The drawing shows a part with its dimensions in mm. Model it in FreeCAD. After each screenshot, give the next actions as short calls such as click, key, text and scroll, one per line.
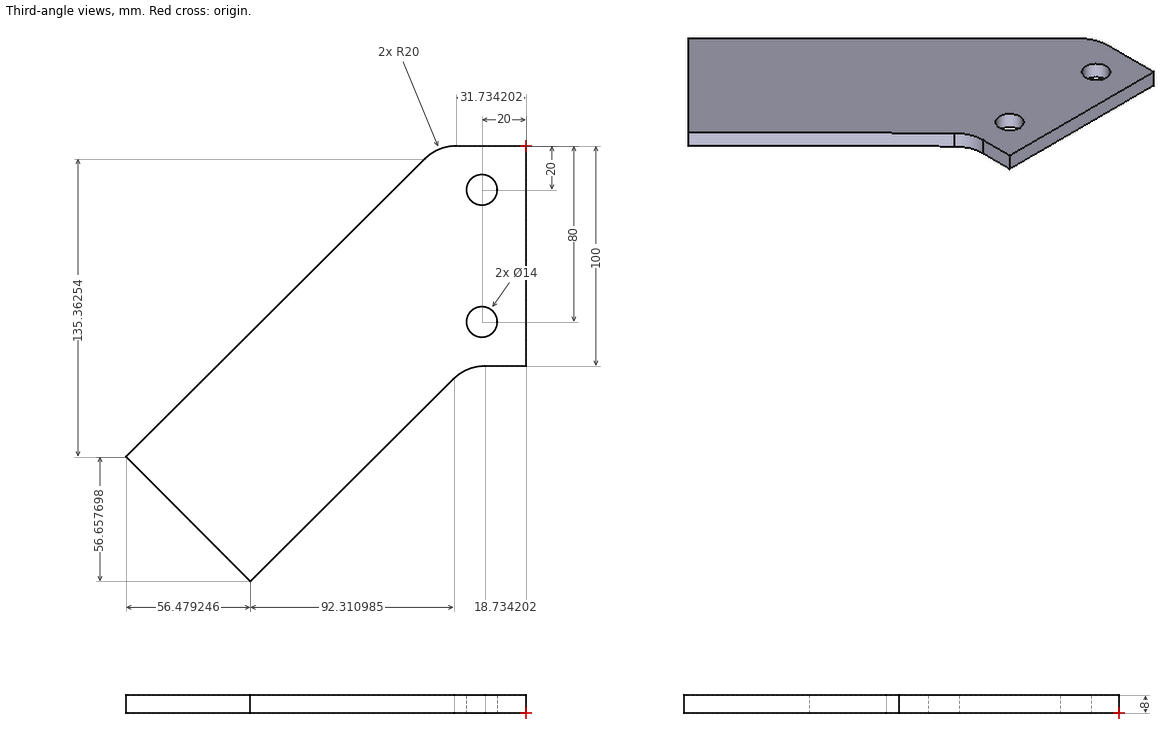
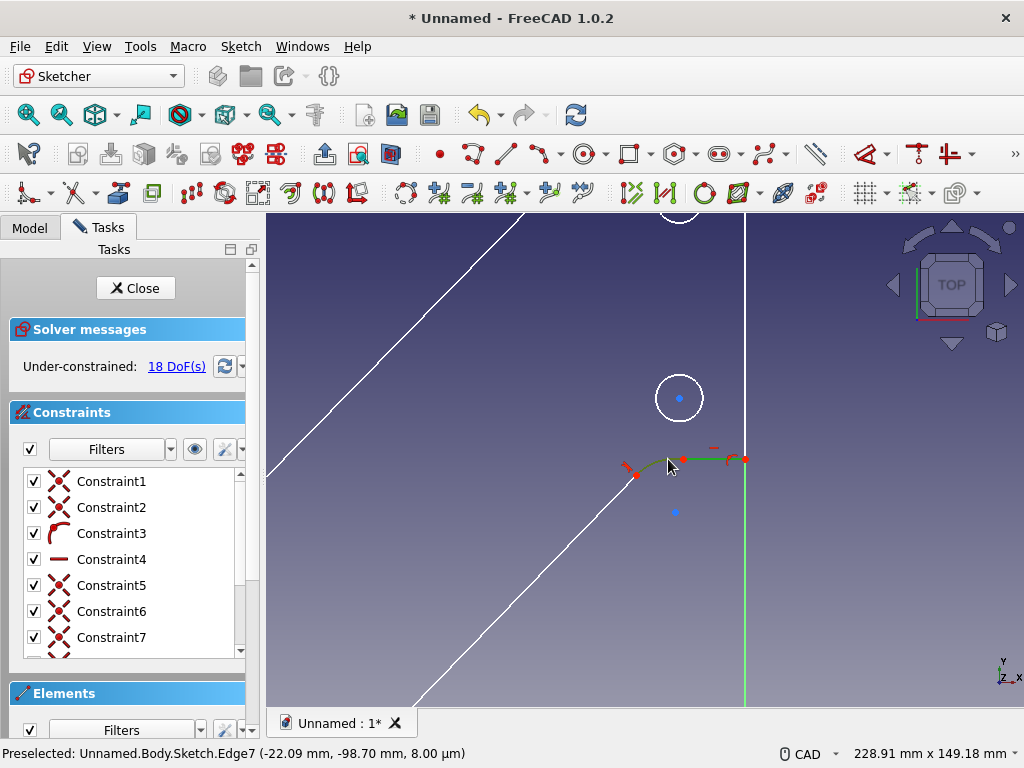
key(t)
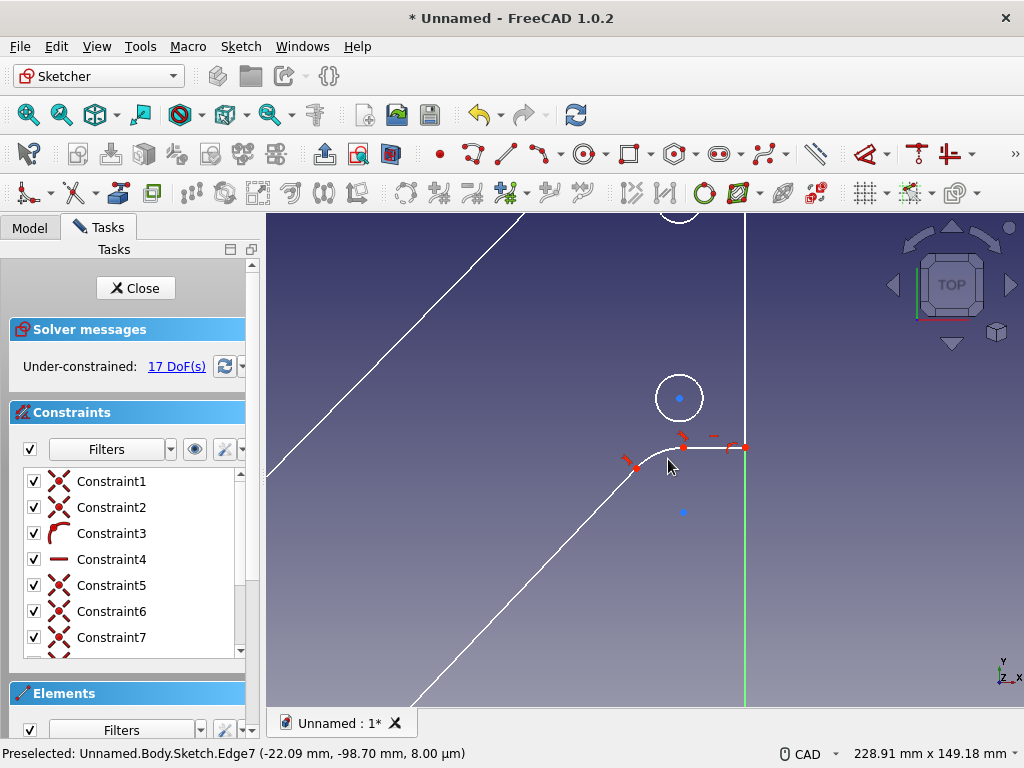
scroll(684, 460, down, 4)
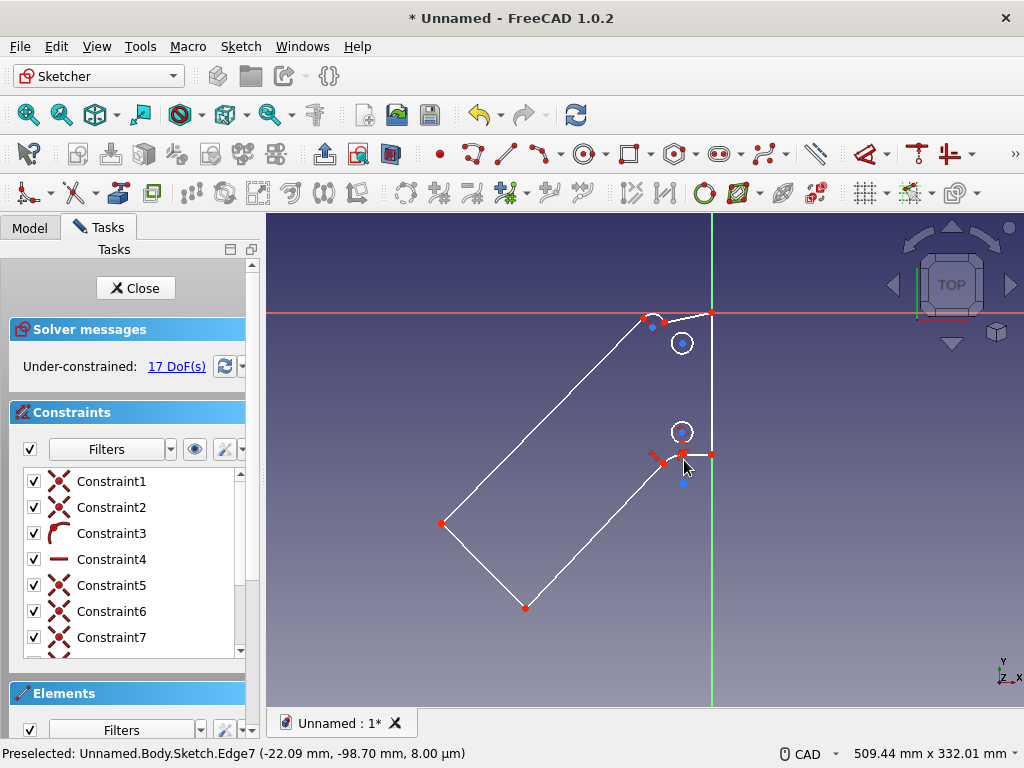
scroll(679, 320, up, 4)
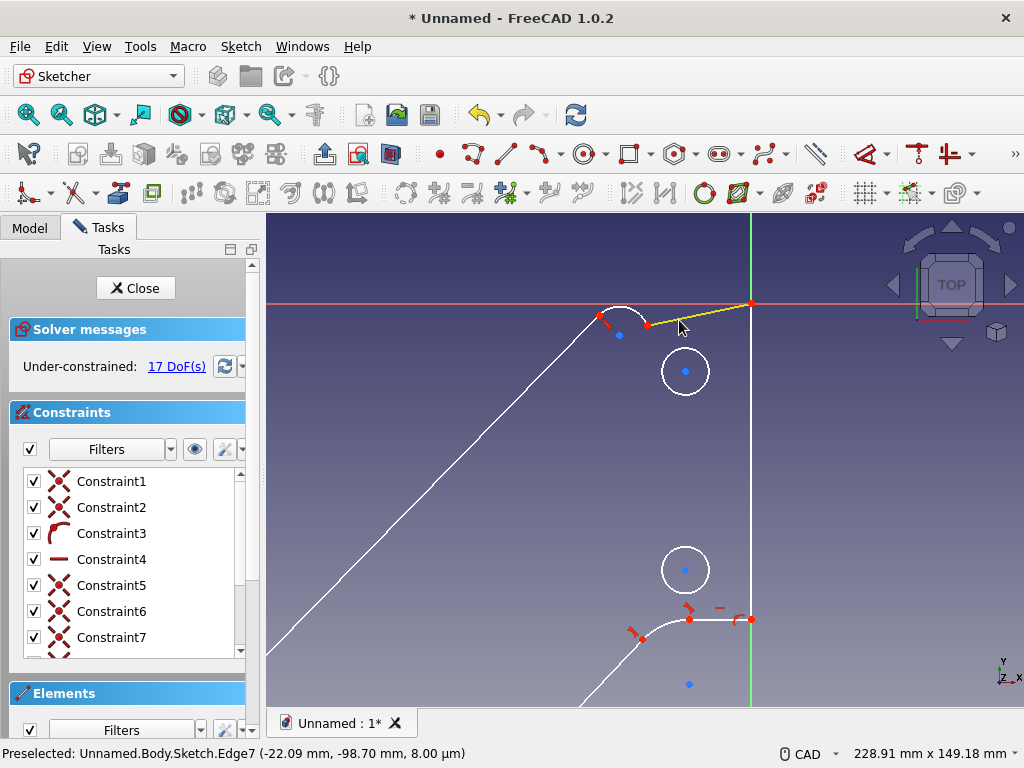
click(678, 319)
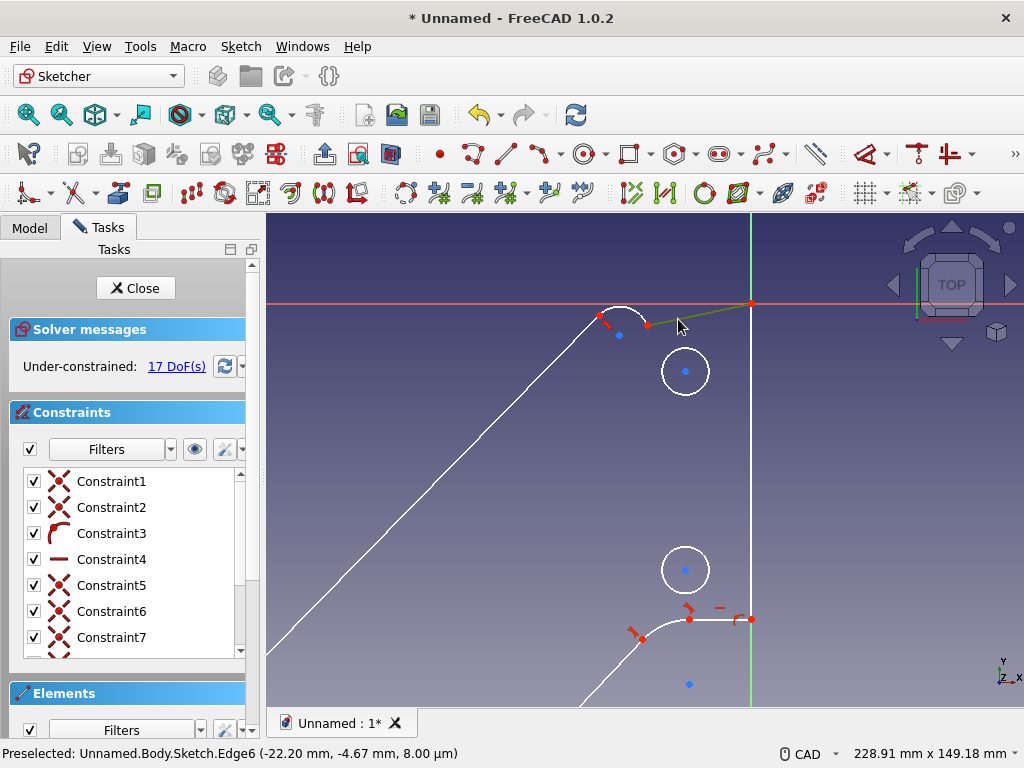
click(614, 307)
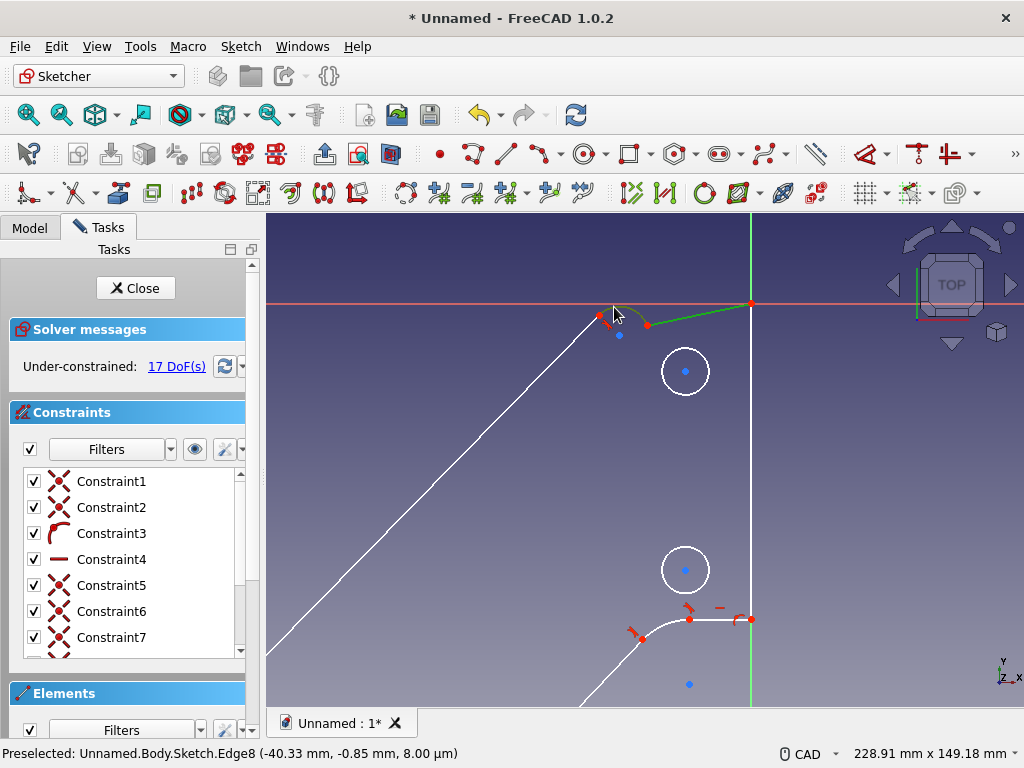
key(t)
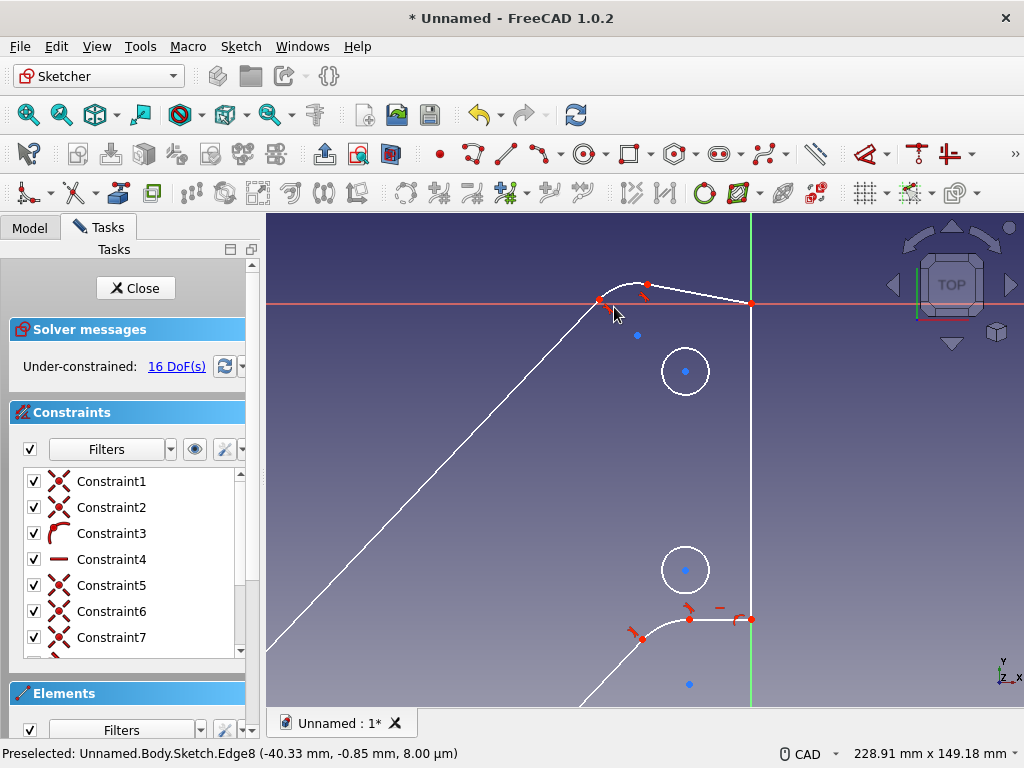
click(678, 290)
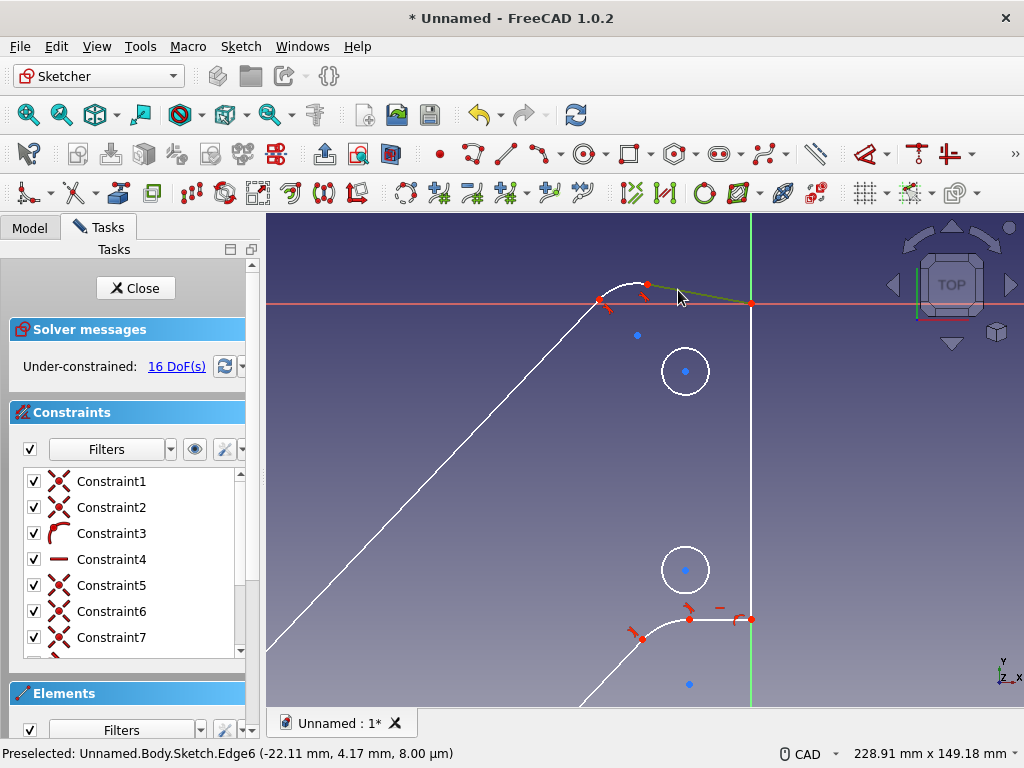
key(h)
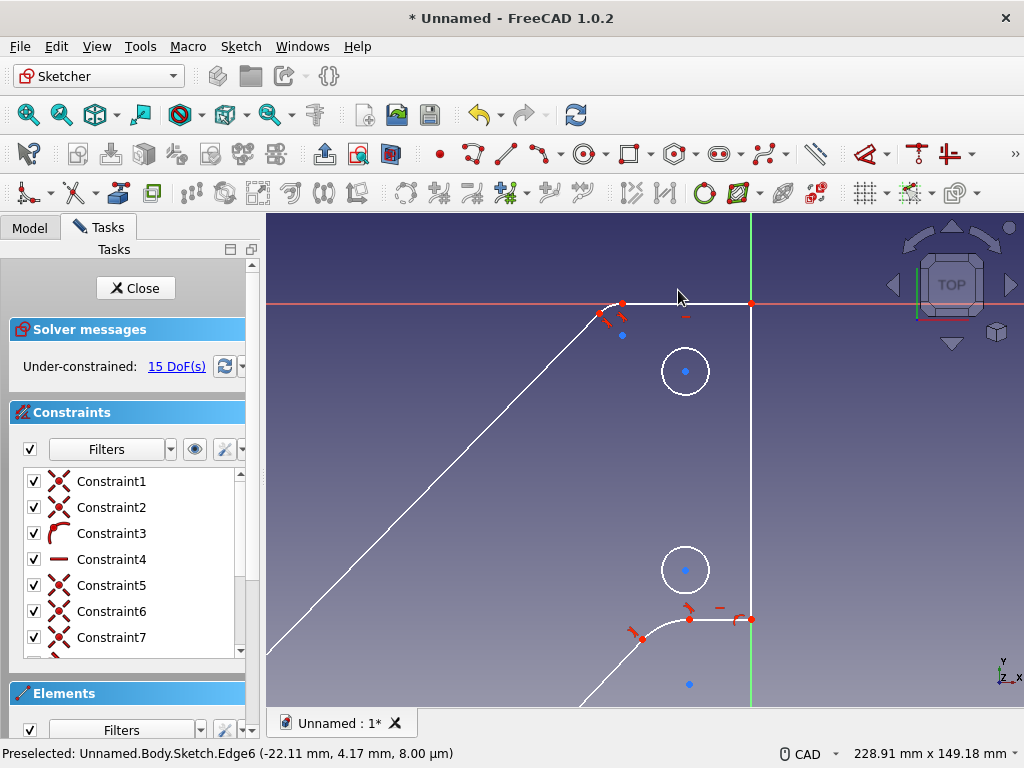
click(674, 622)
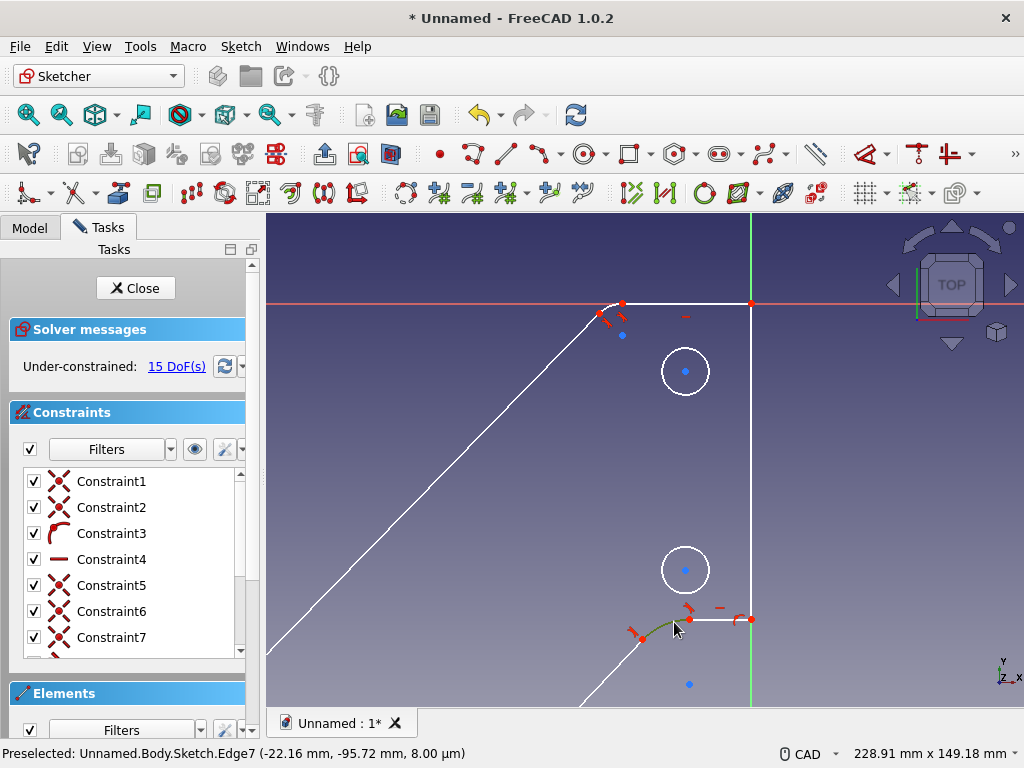
click(610, 306)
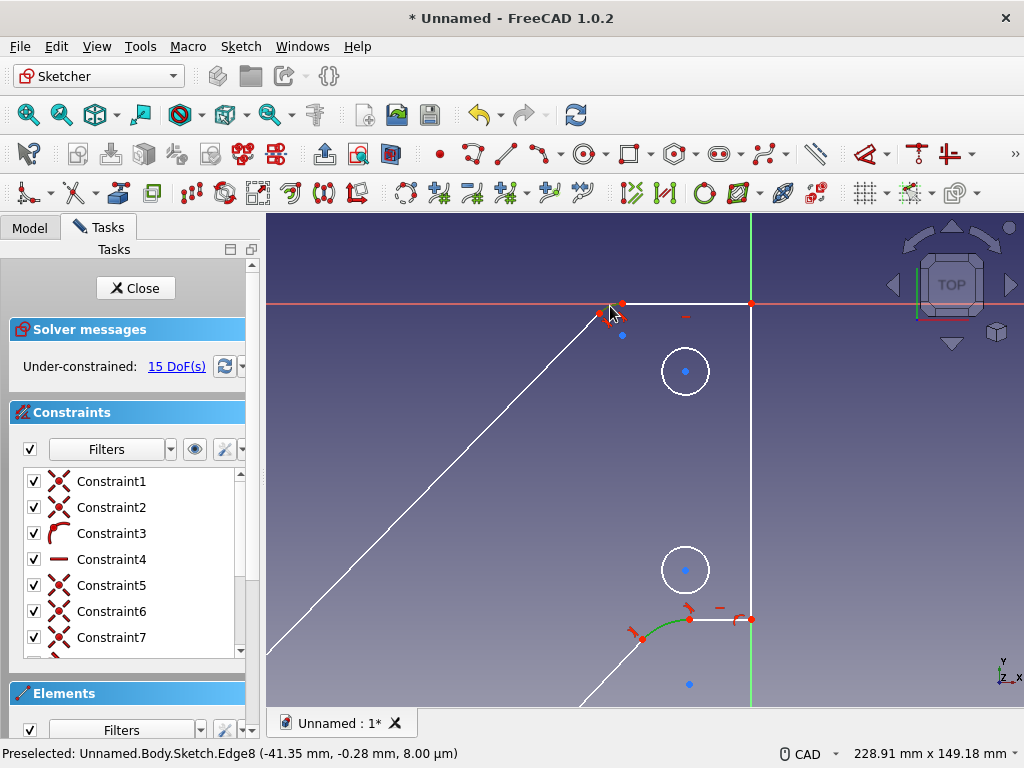
key(e)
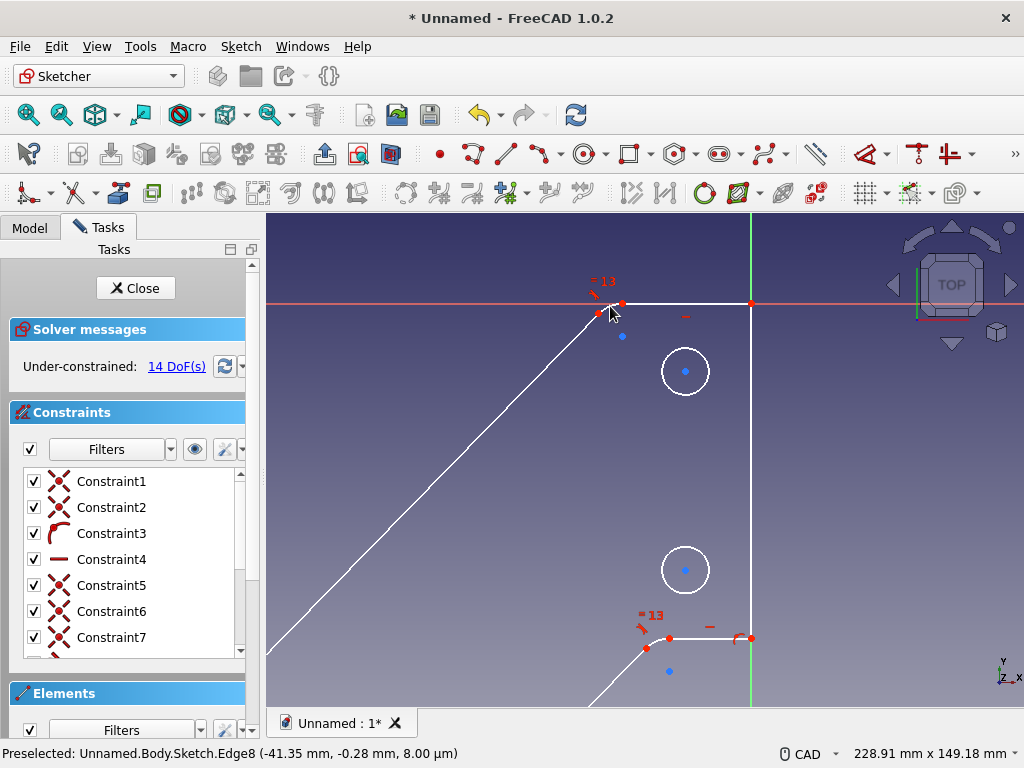
click(702, 553)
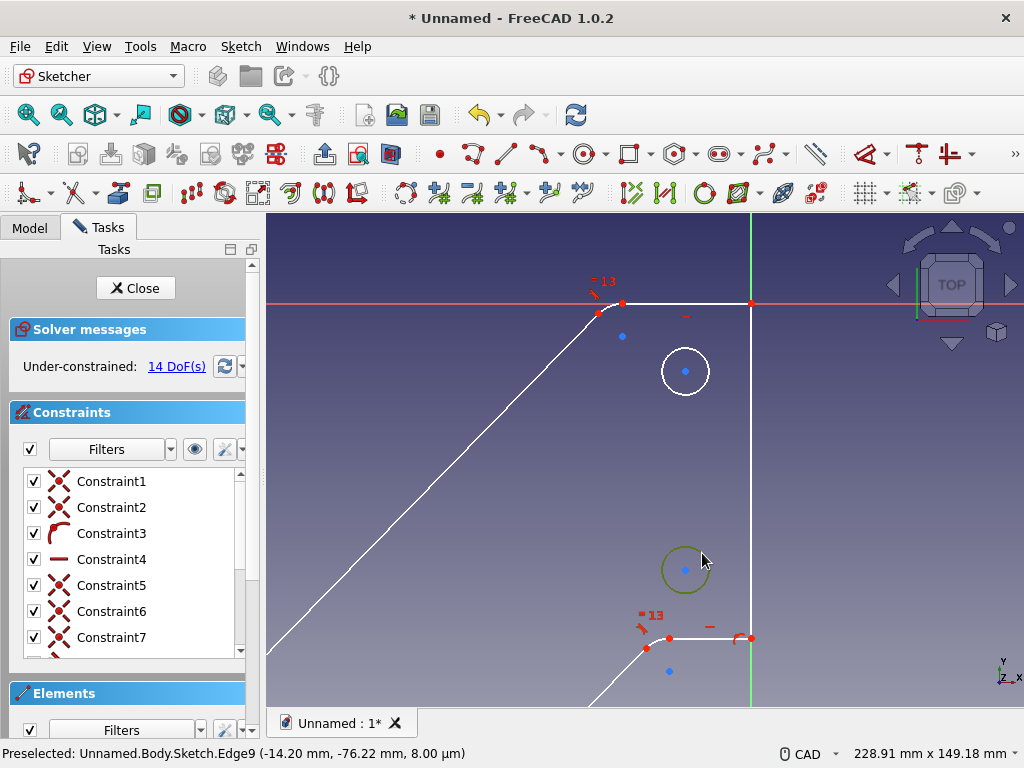
click(702, 355)